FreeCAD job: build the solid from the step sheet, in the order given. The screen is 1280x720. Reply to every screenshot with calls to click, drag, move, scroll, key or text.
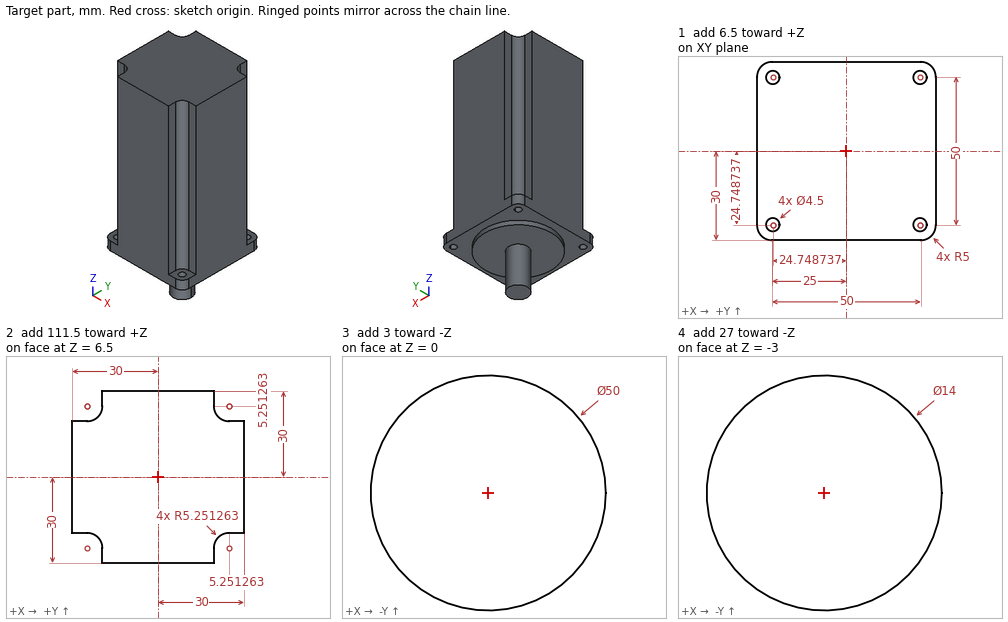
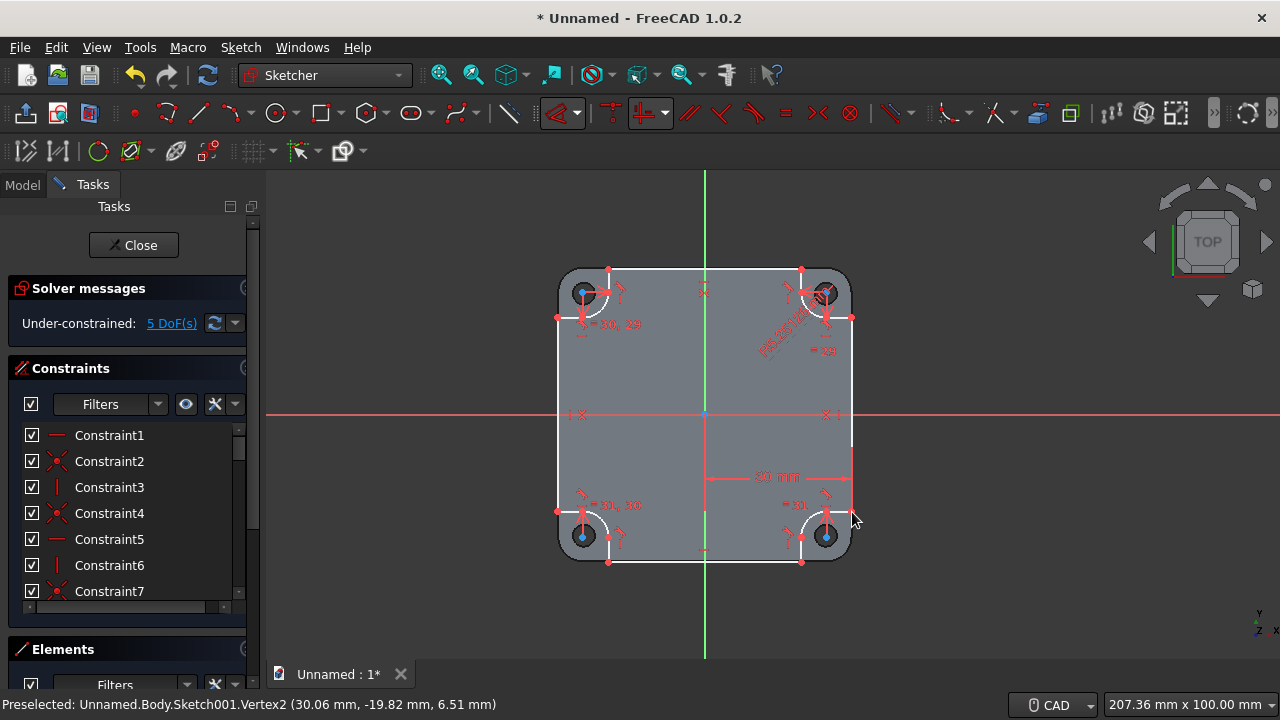
click(801, 269)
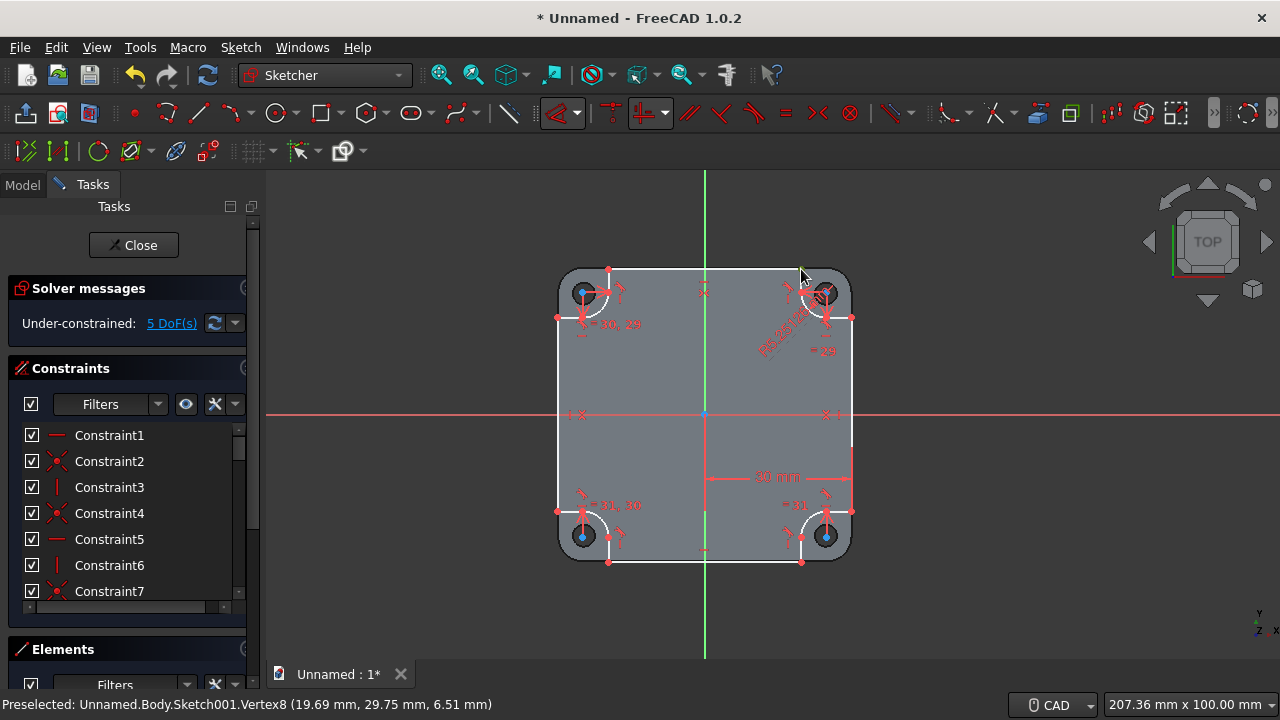
key(i)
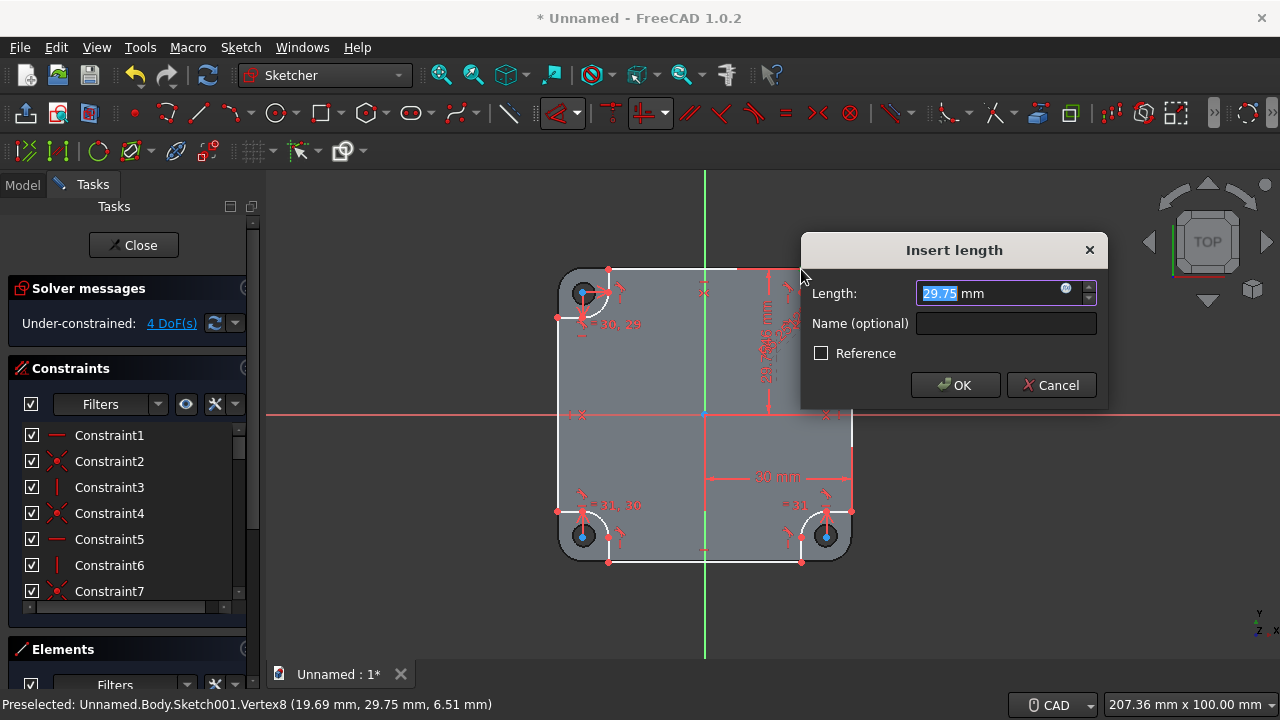
text(30)
key(Return)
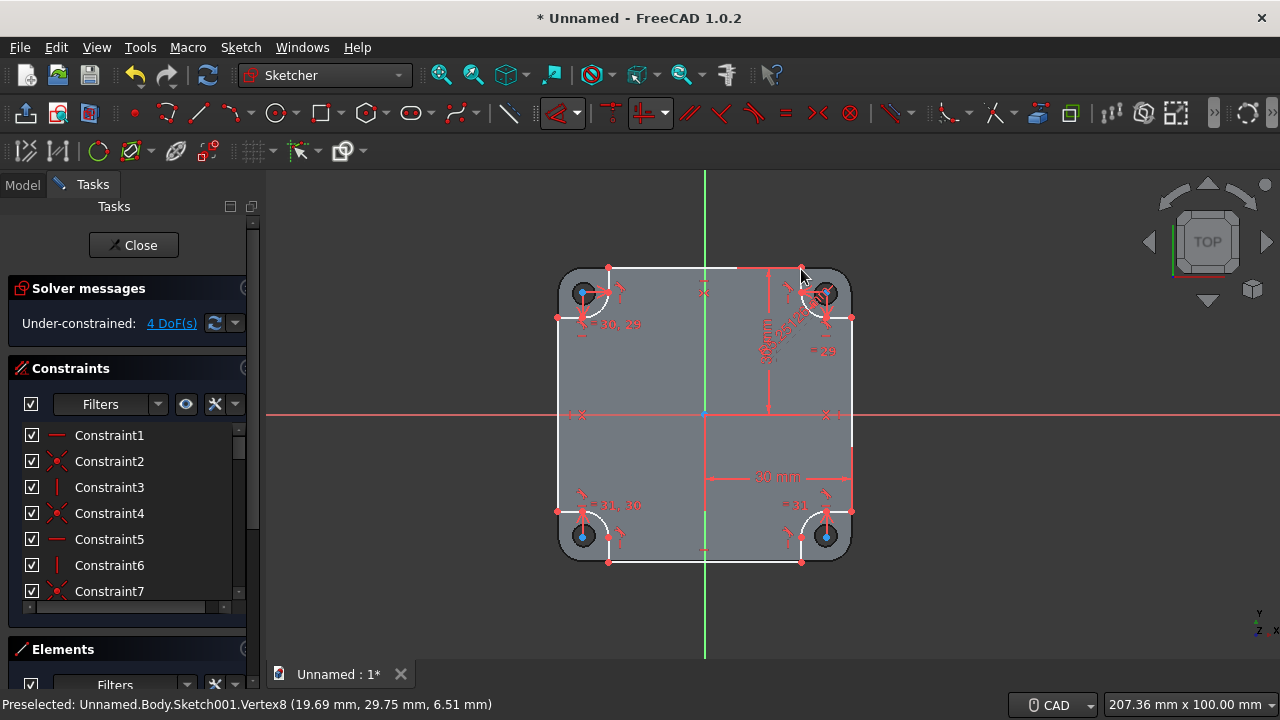
click(558, 318)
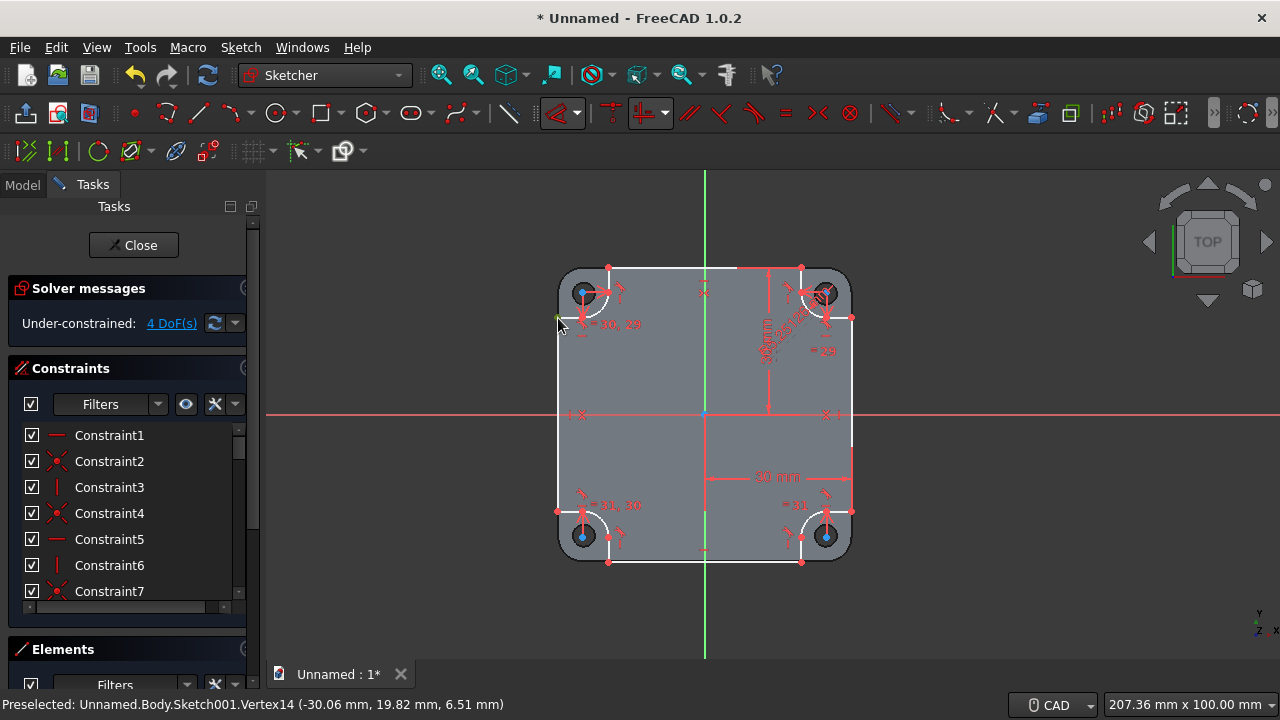
key(l)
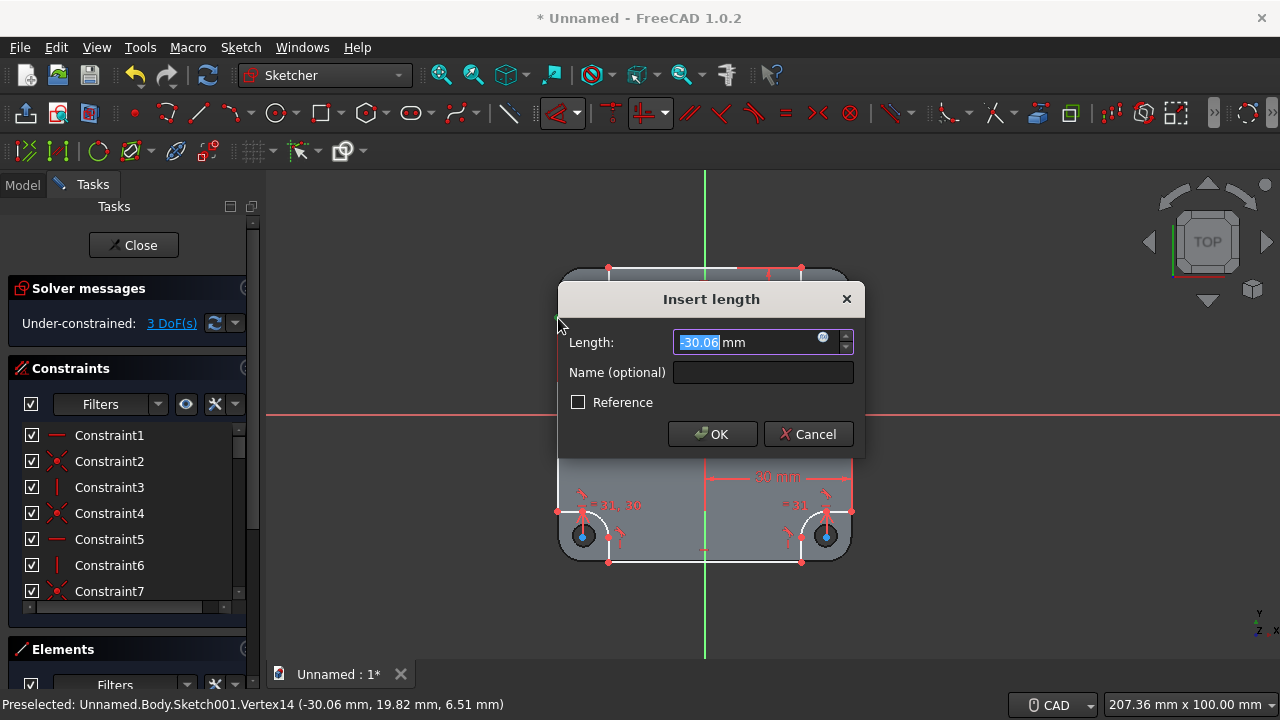
text(-30)
key(Return)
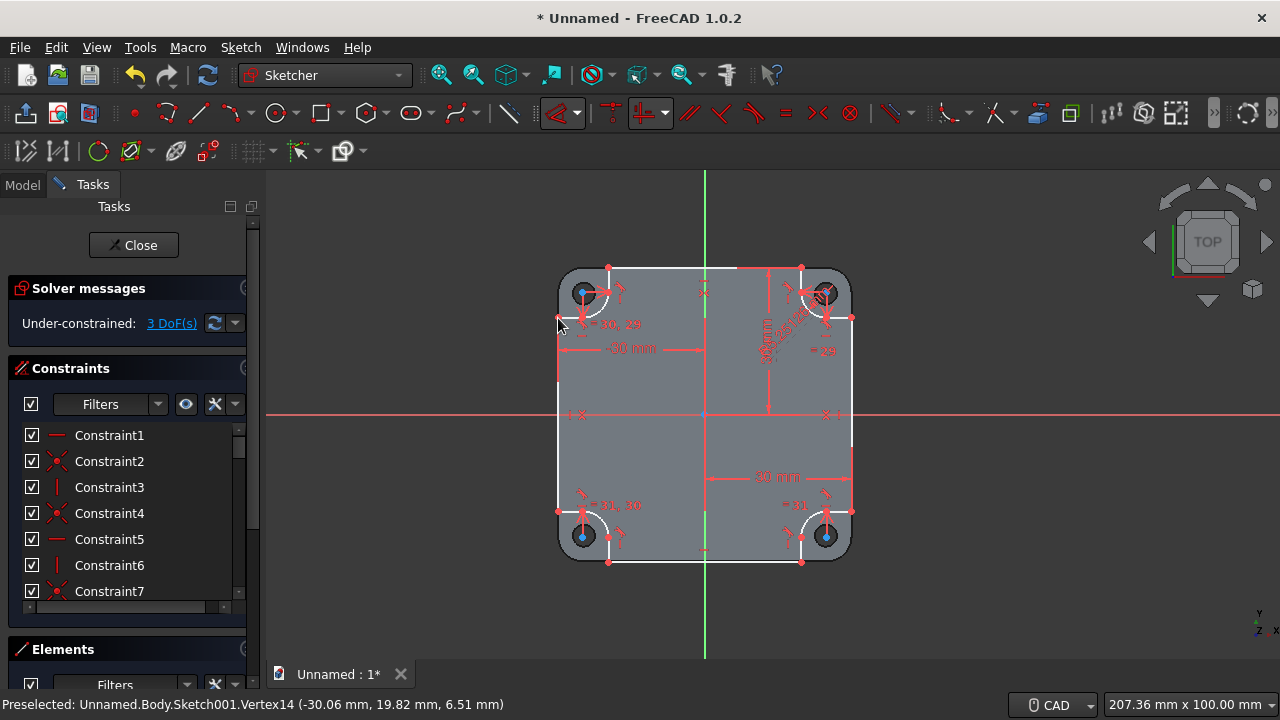
click(609, 562)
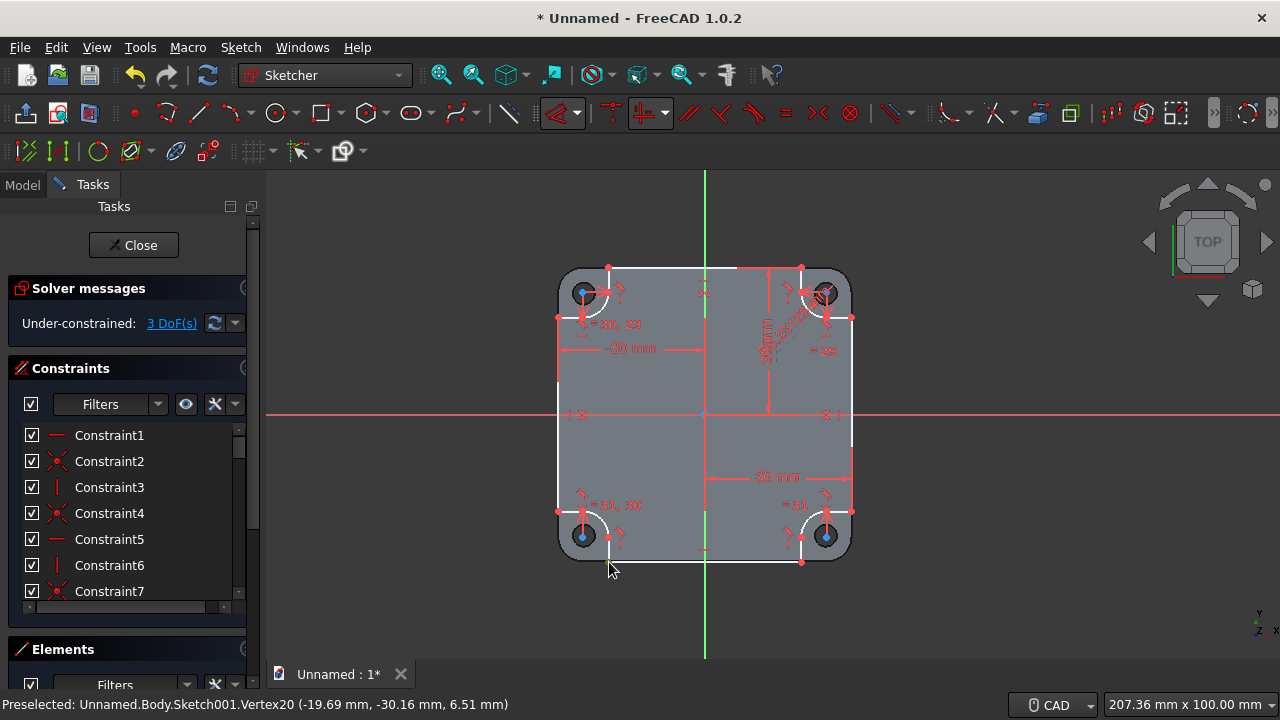
click(580, 114)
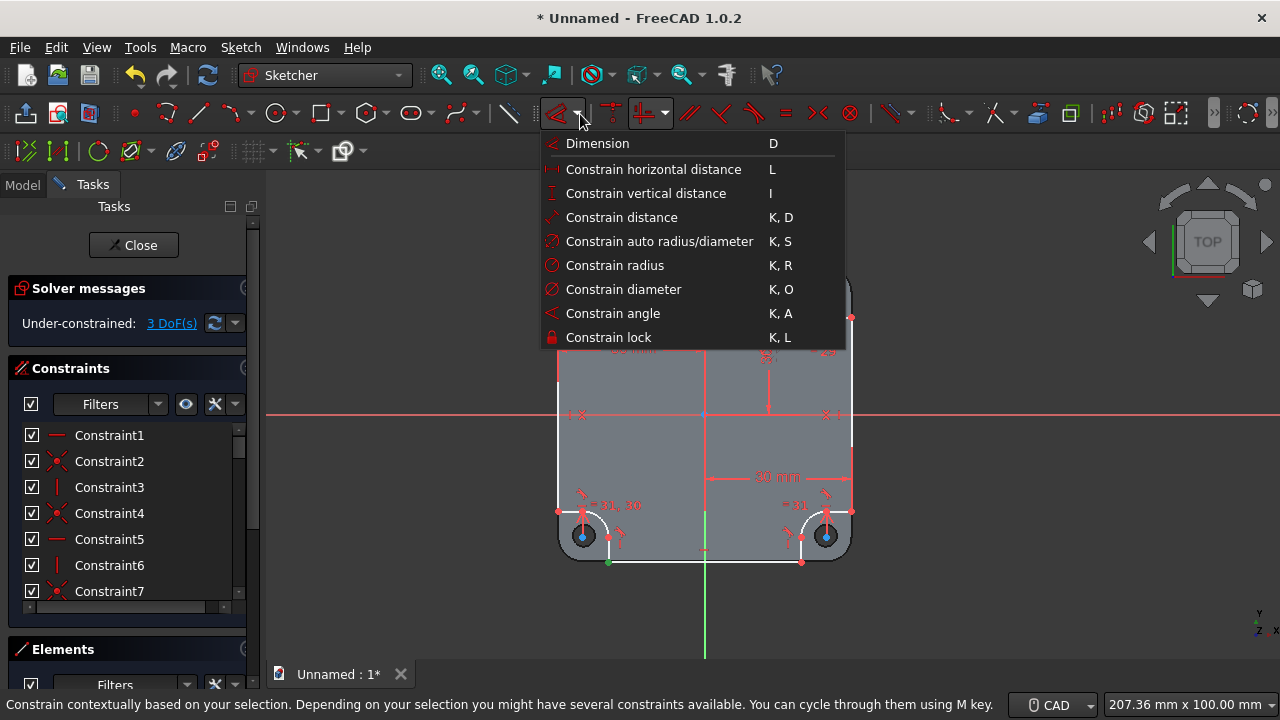
click(693, 193)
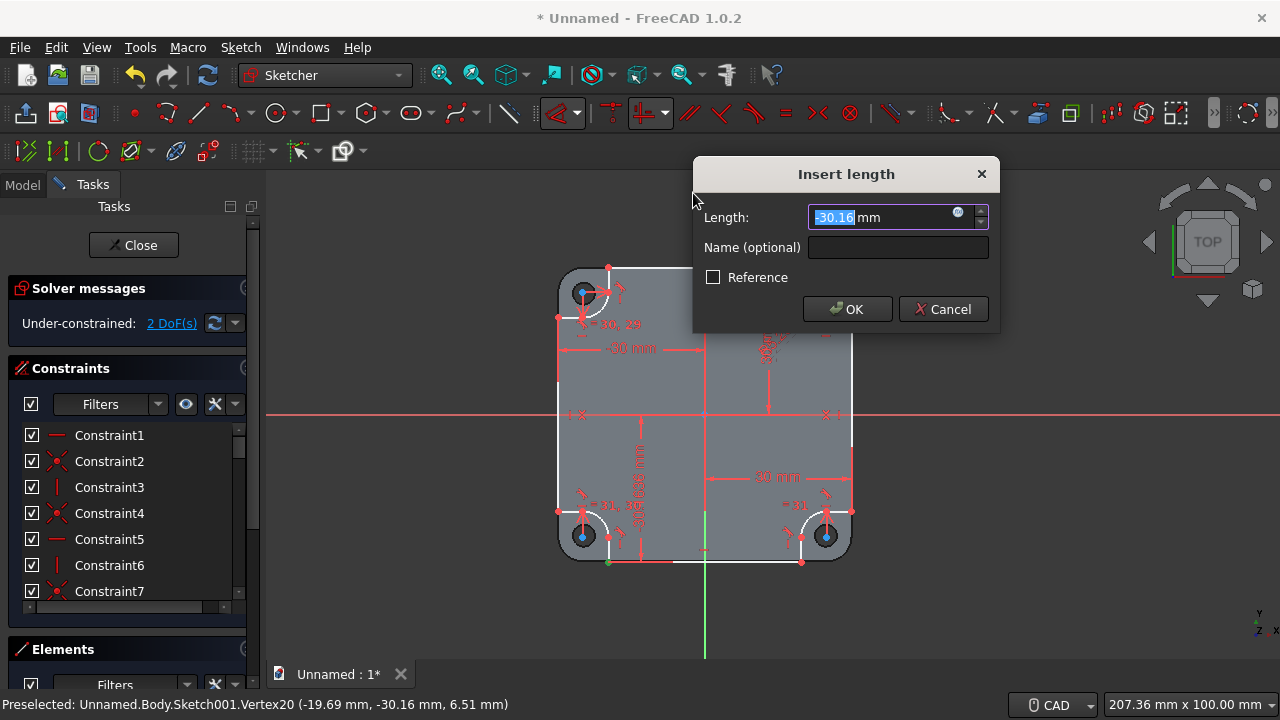
text(-30)
key(Return)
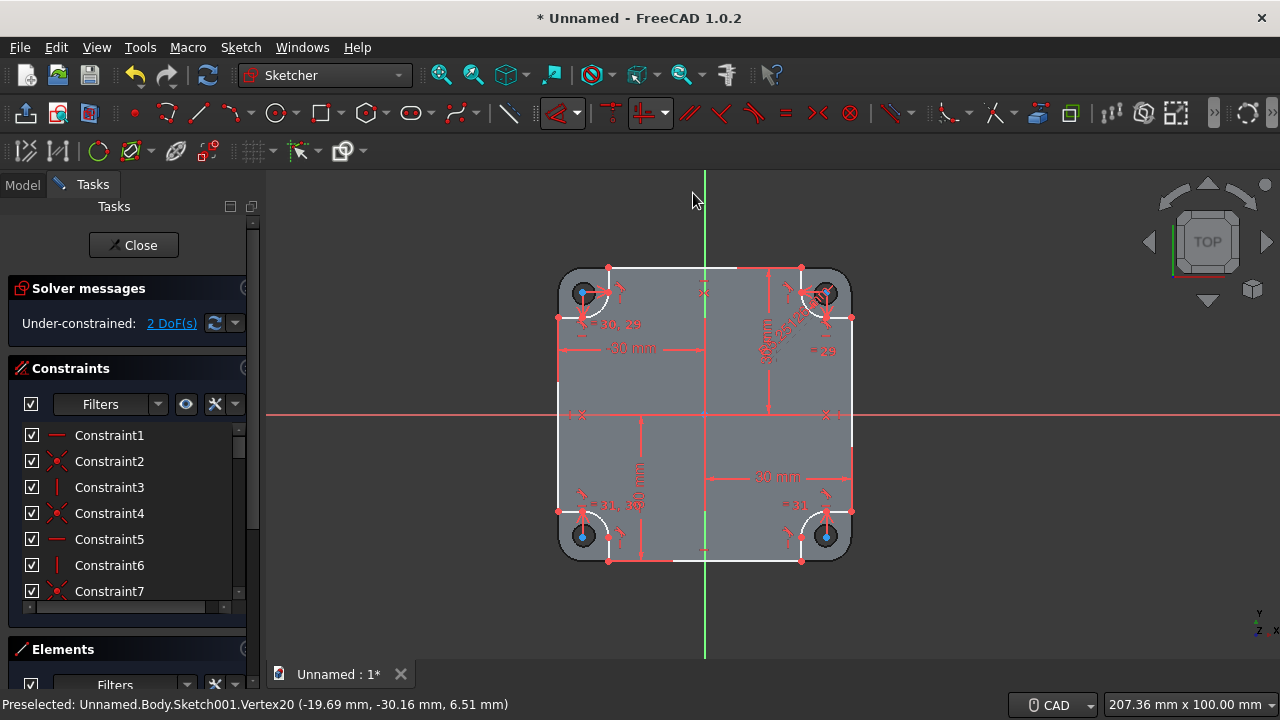
scroll(837, 512, up, 3)